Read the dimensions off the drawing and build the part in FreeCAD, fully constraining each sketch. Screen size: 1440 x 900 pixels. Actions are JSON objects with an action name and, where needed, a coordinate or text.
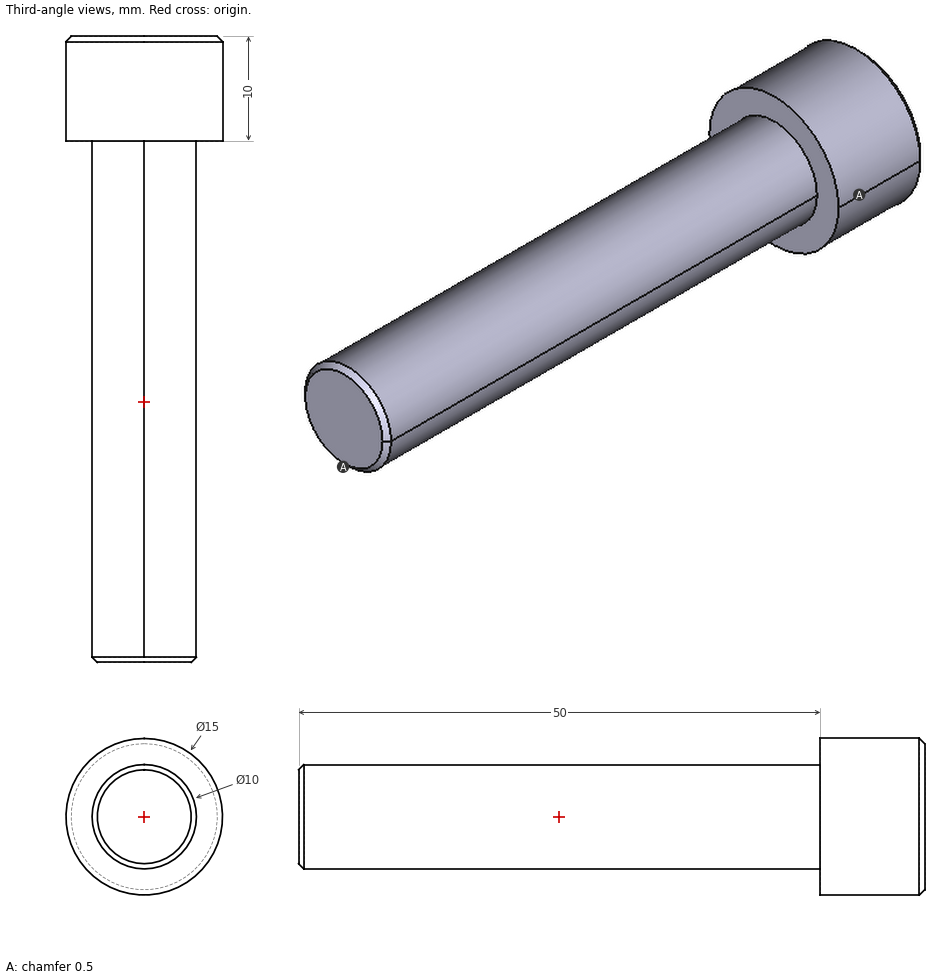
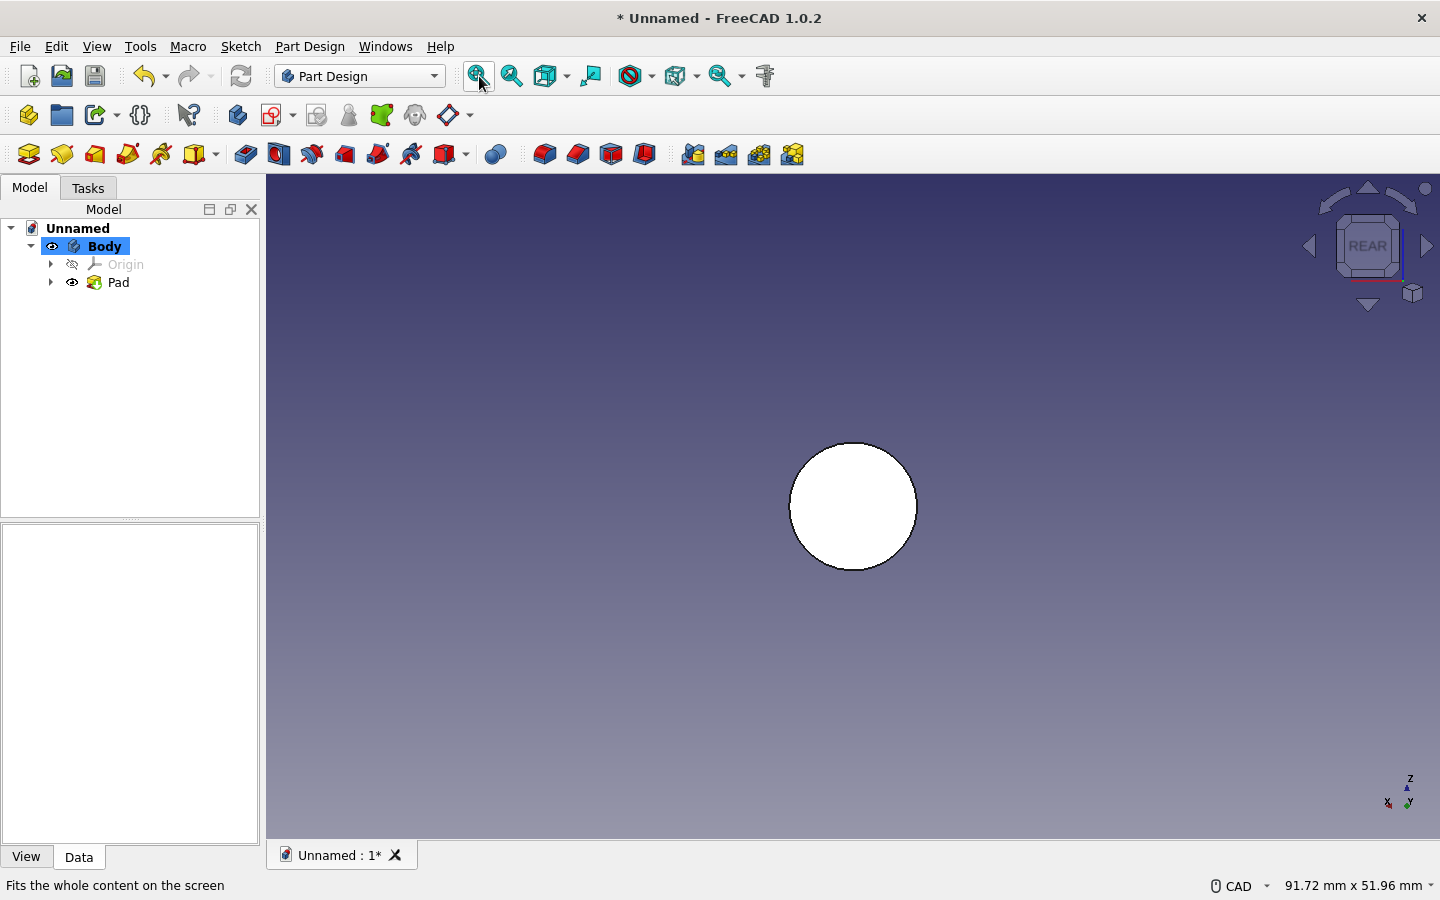
{"action": "left_click", "coordinate": [479, 76]}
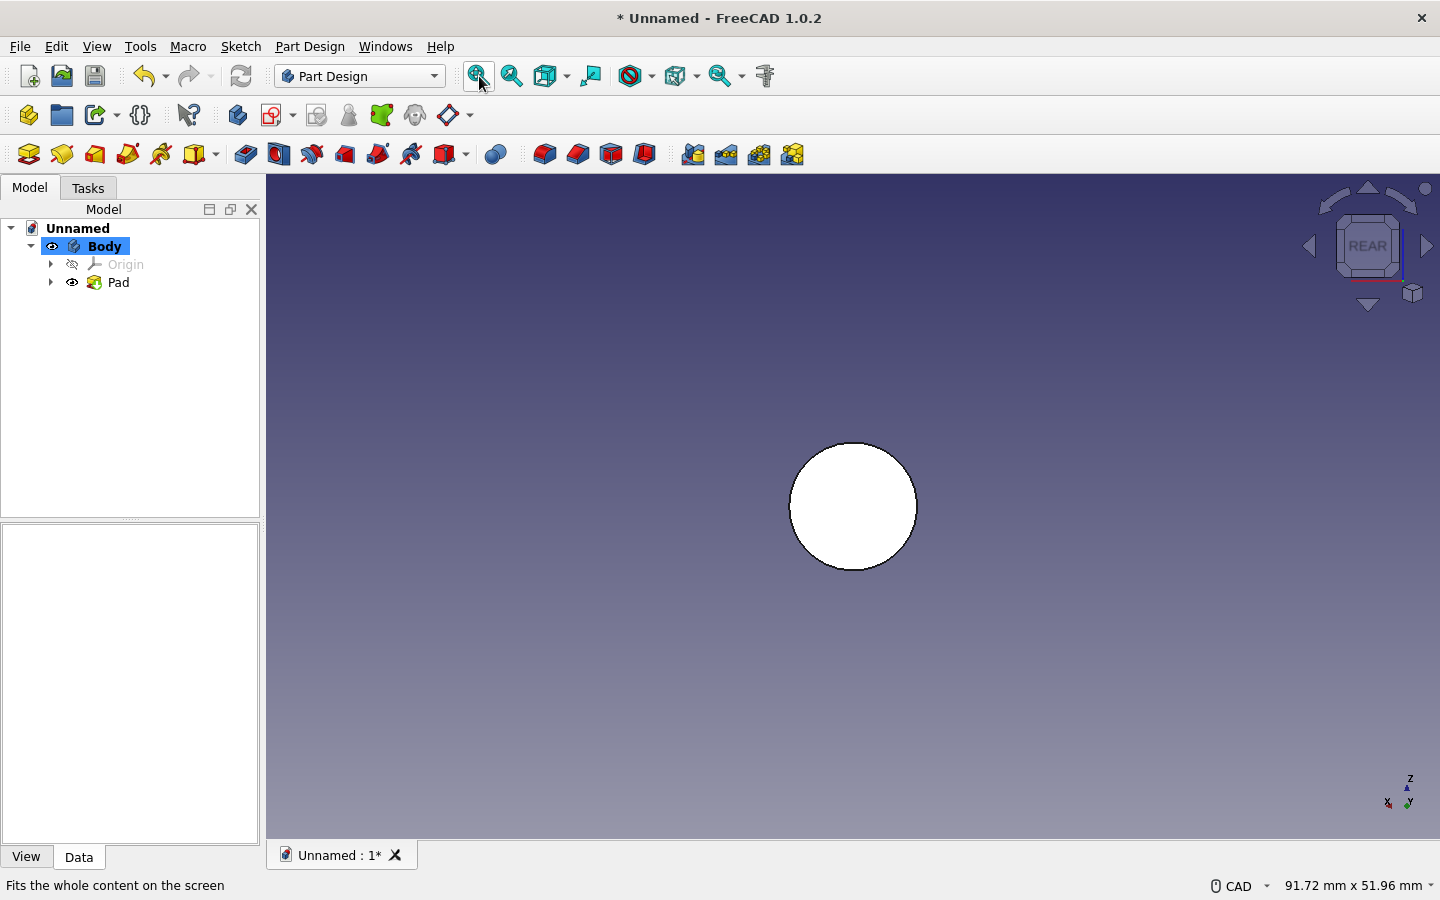
{"action": "left_click", "coordinate": [853, 506]}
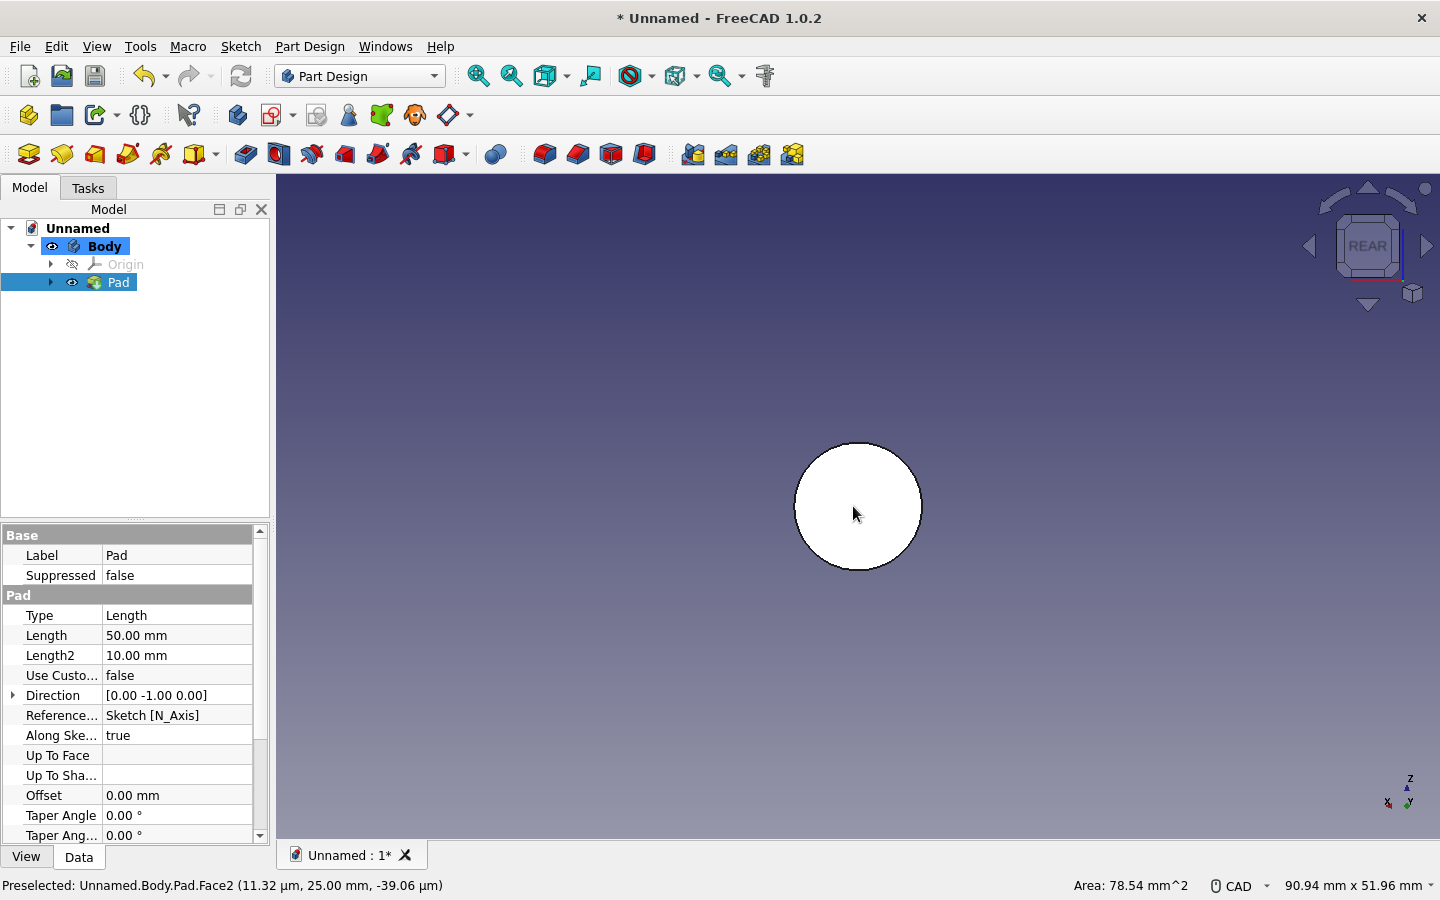
{"action": "left_click", "coordinate": [270, 116]}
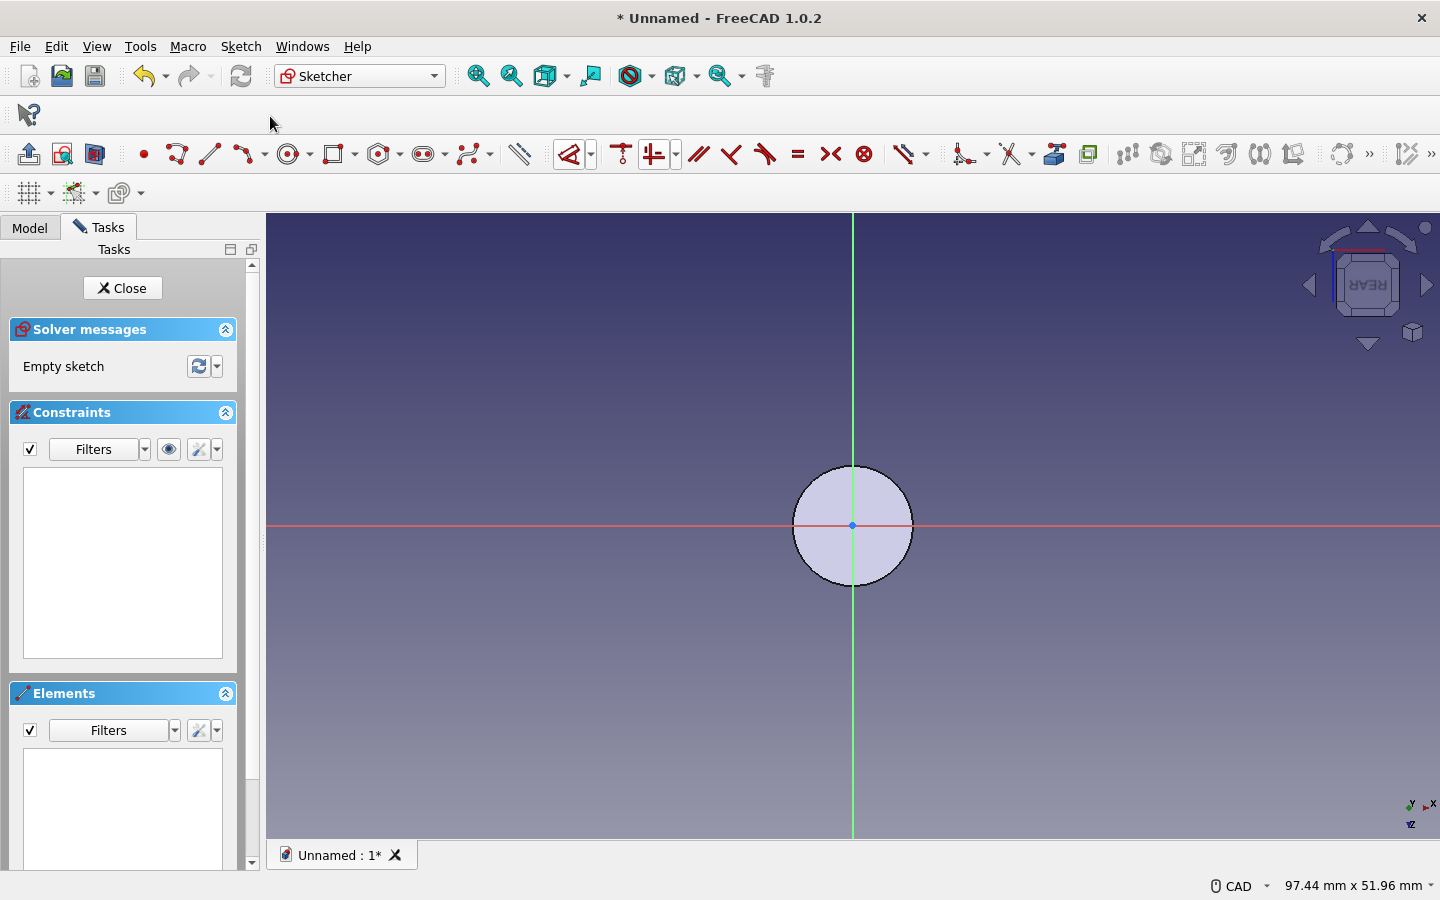
{"action": "scroll", "coordinate": [909, 526], "scroll_direction": "up", "scroll_amount": 4}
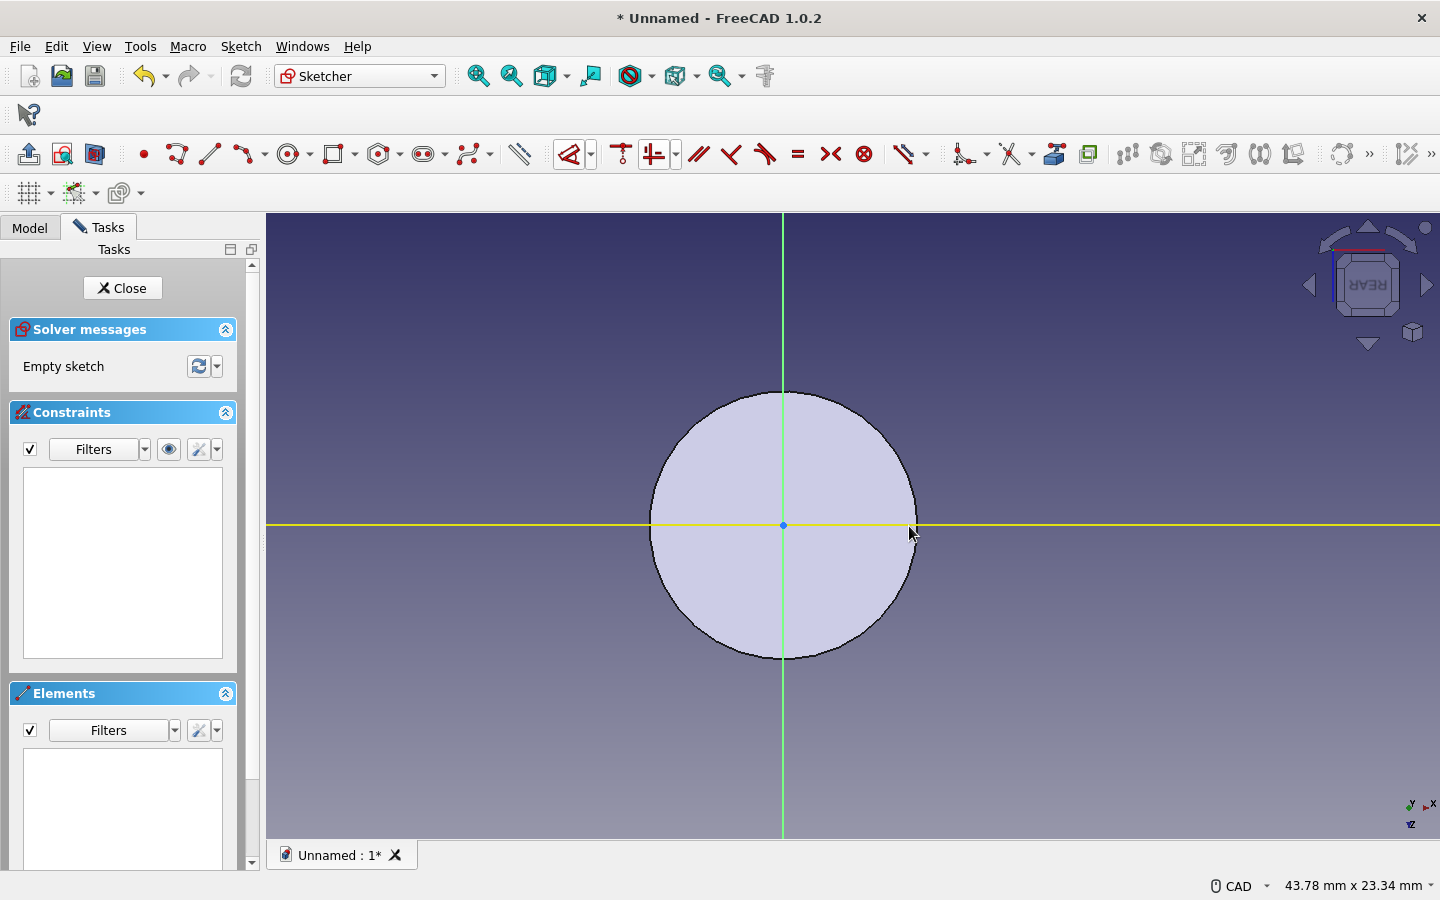
{"action": "left_click", "coordinate": [288, 154]}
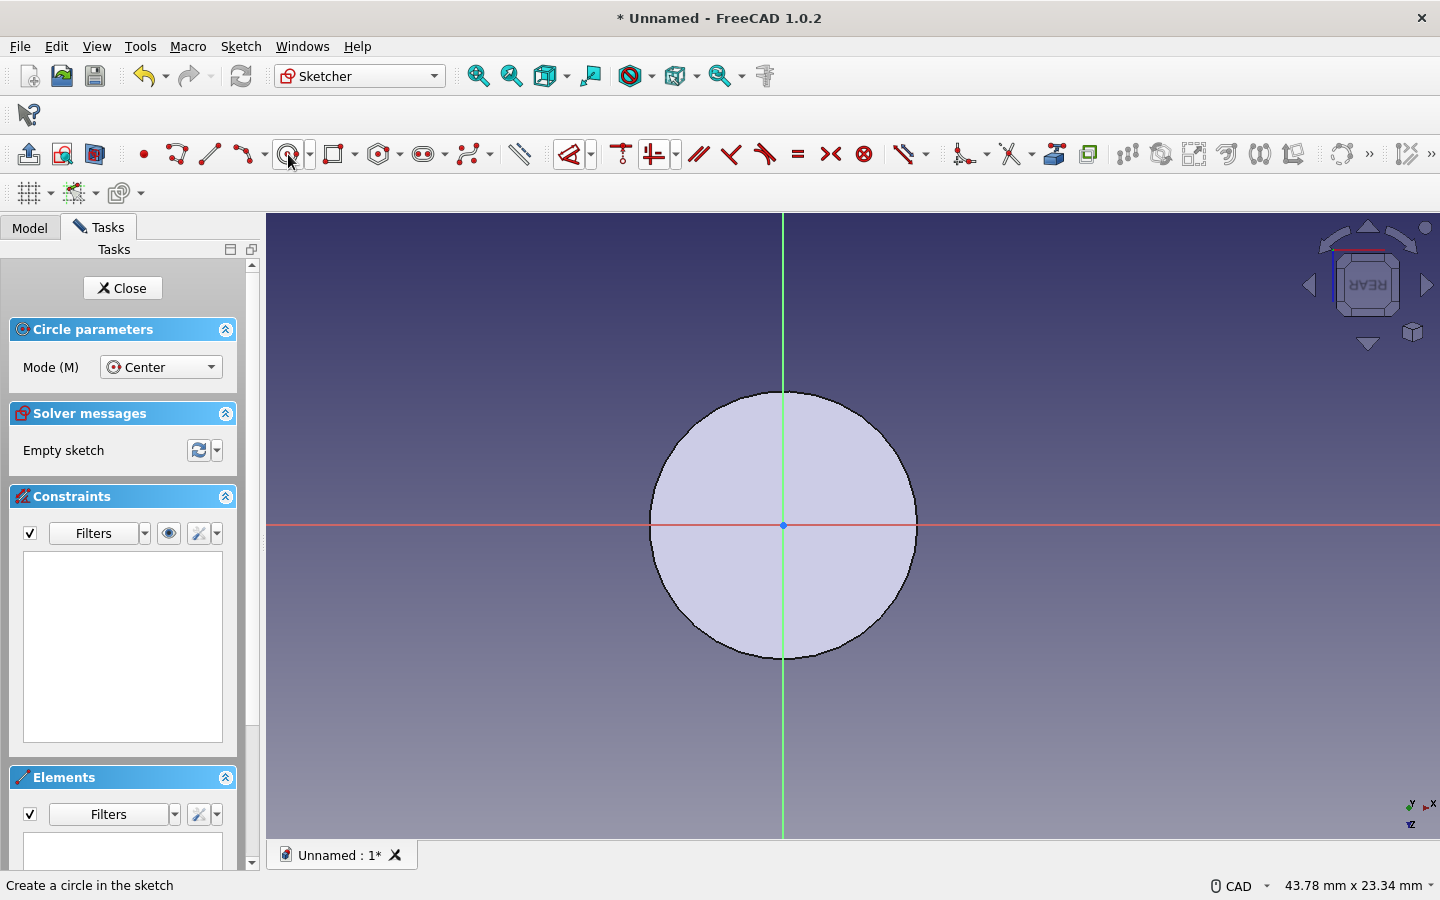
{"action": "left_click", "coordinate": [783, 525]}
{"action": "mouse_move", "coordinate": [926, 383]}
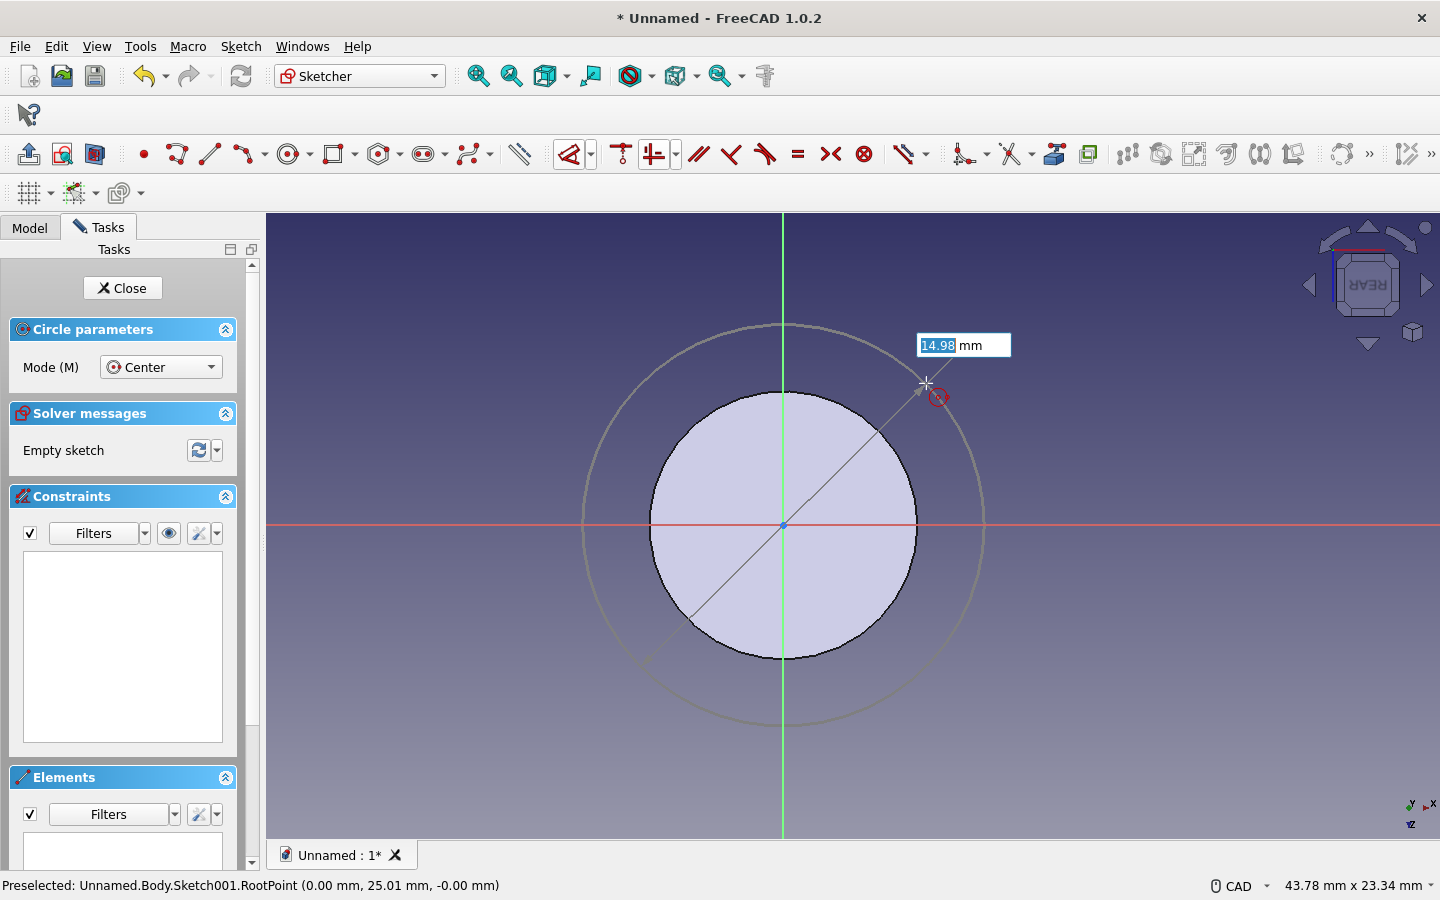
{"action": "type", "text": "15"}
{"action": "key", "text": "Return"}
{"action": "key", "text": "Escape"}